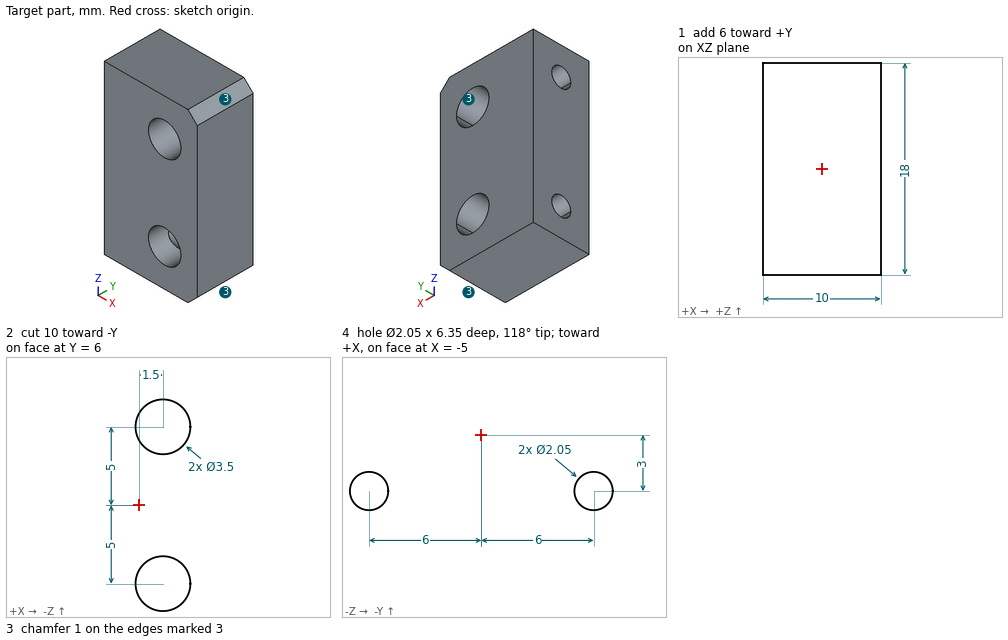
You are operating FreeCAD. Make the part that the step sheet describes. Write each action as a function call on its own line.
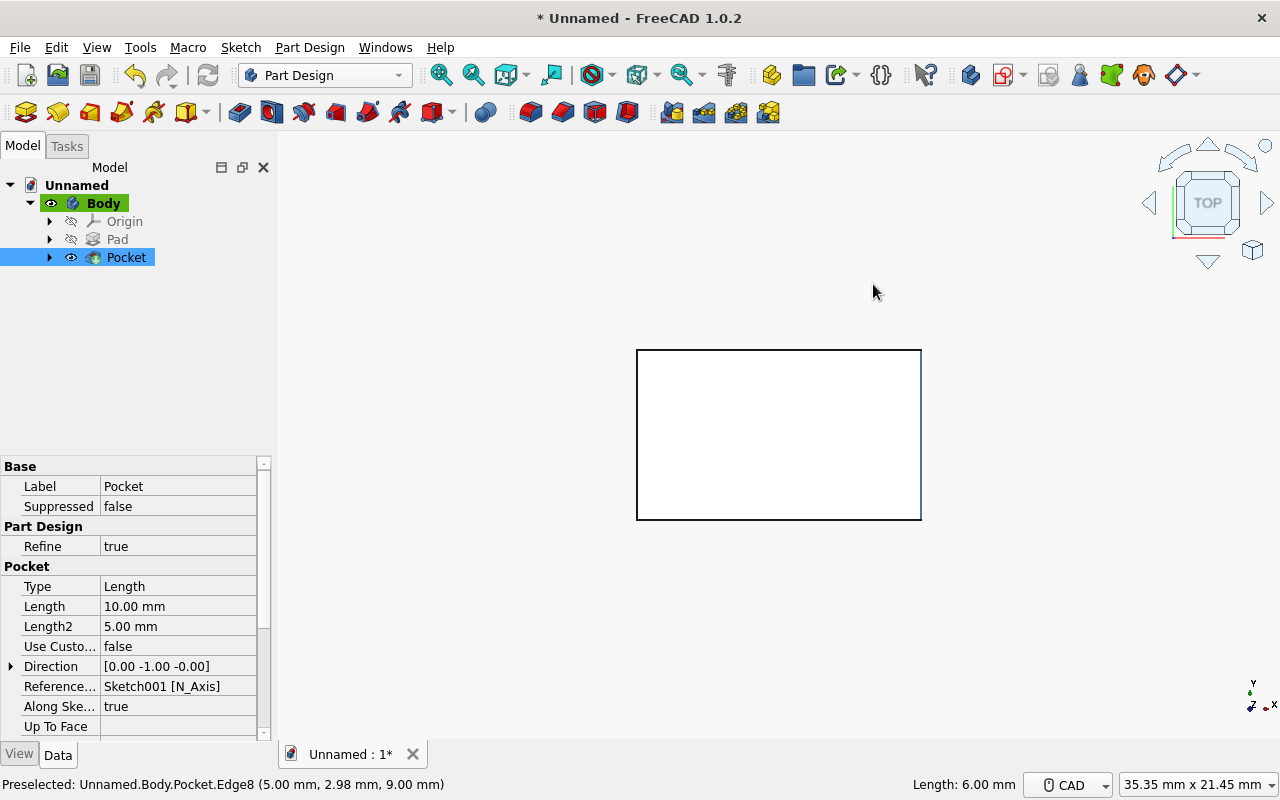
key(1)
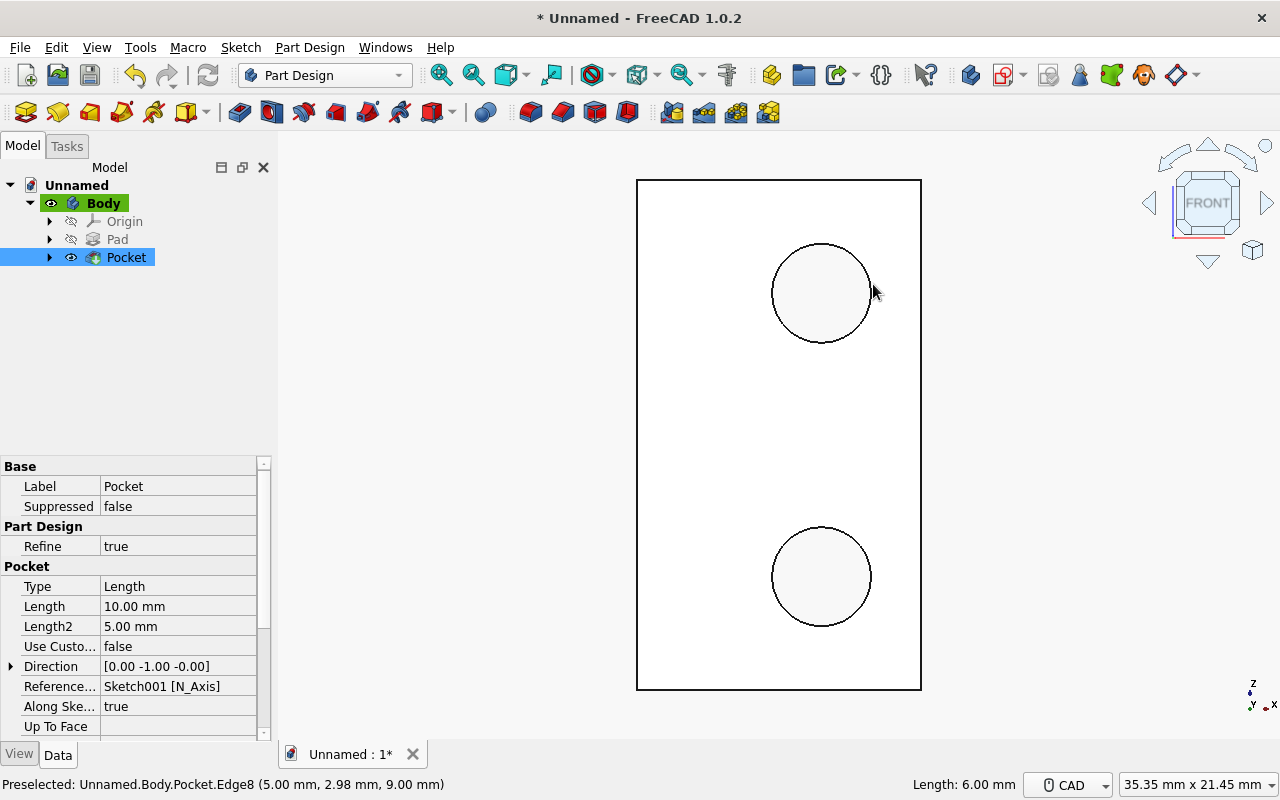
key(3)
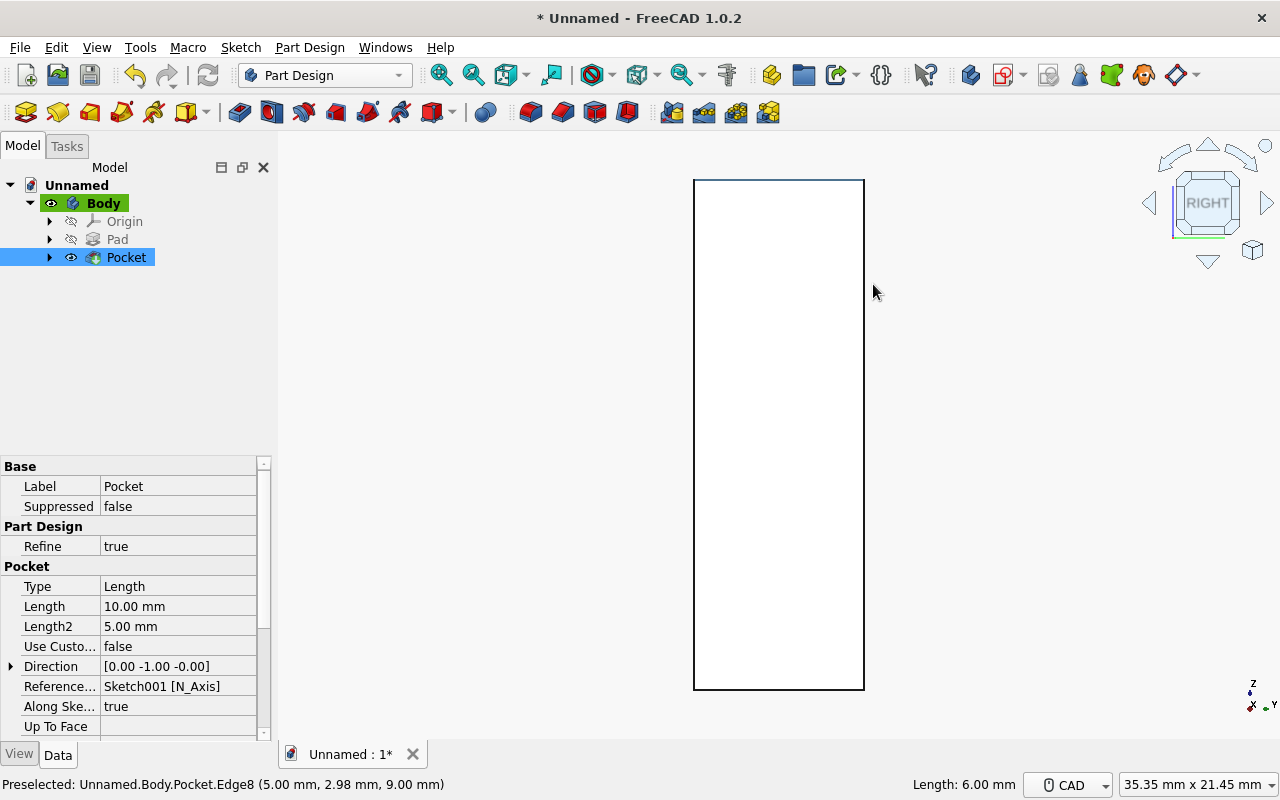
click(779, 689, ctrl)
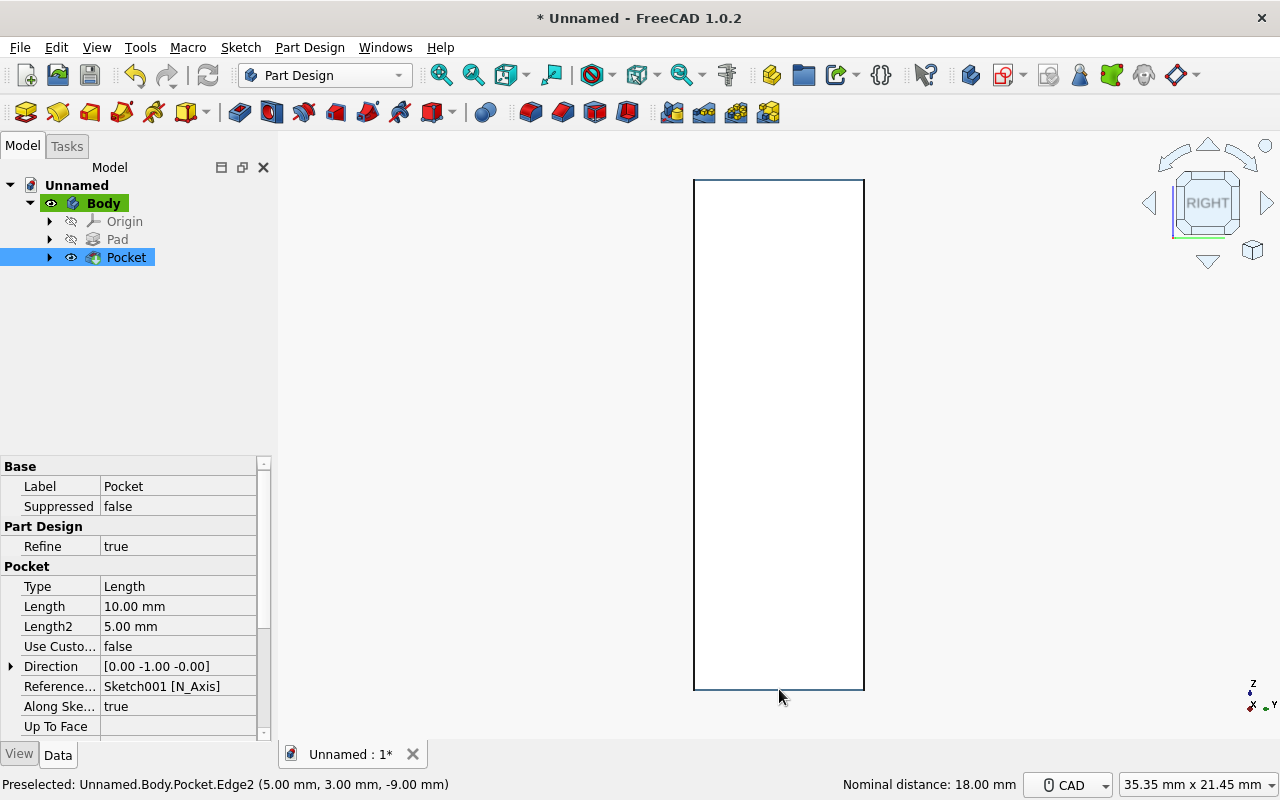
click(564, 112)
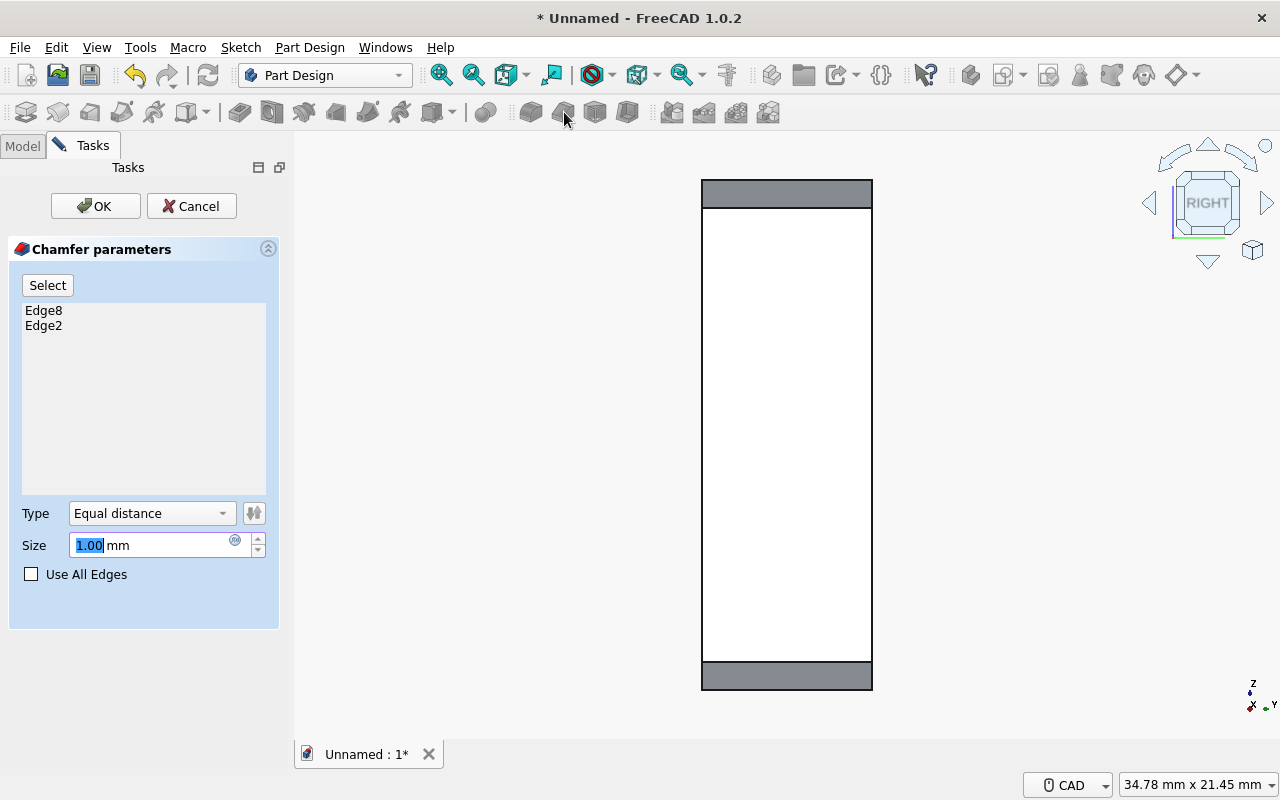
text(1)
key(Tab)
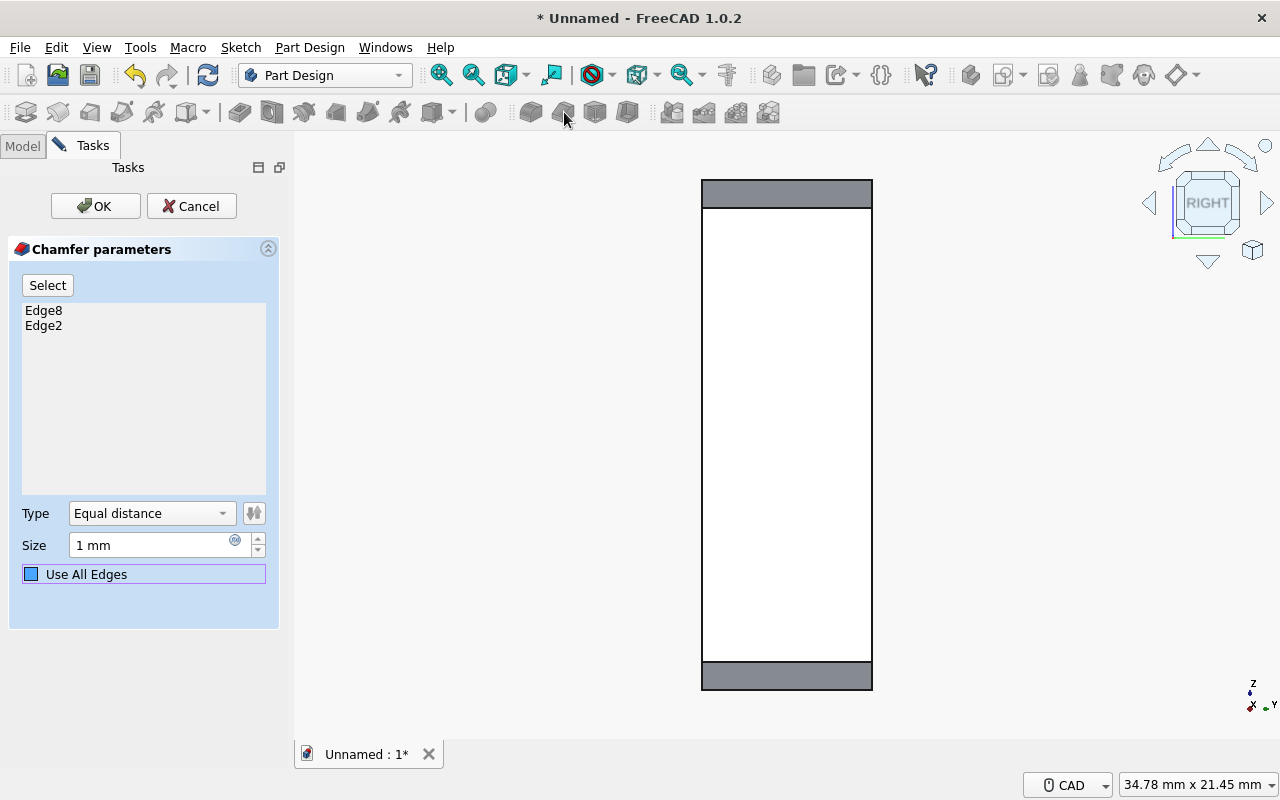
click(96, 206)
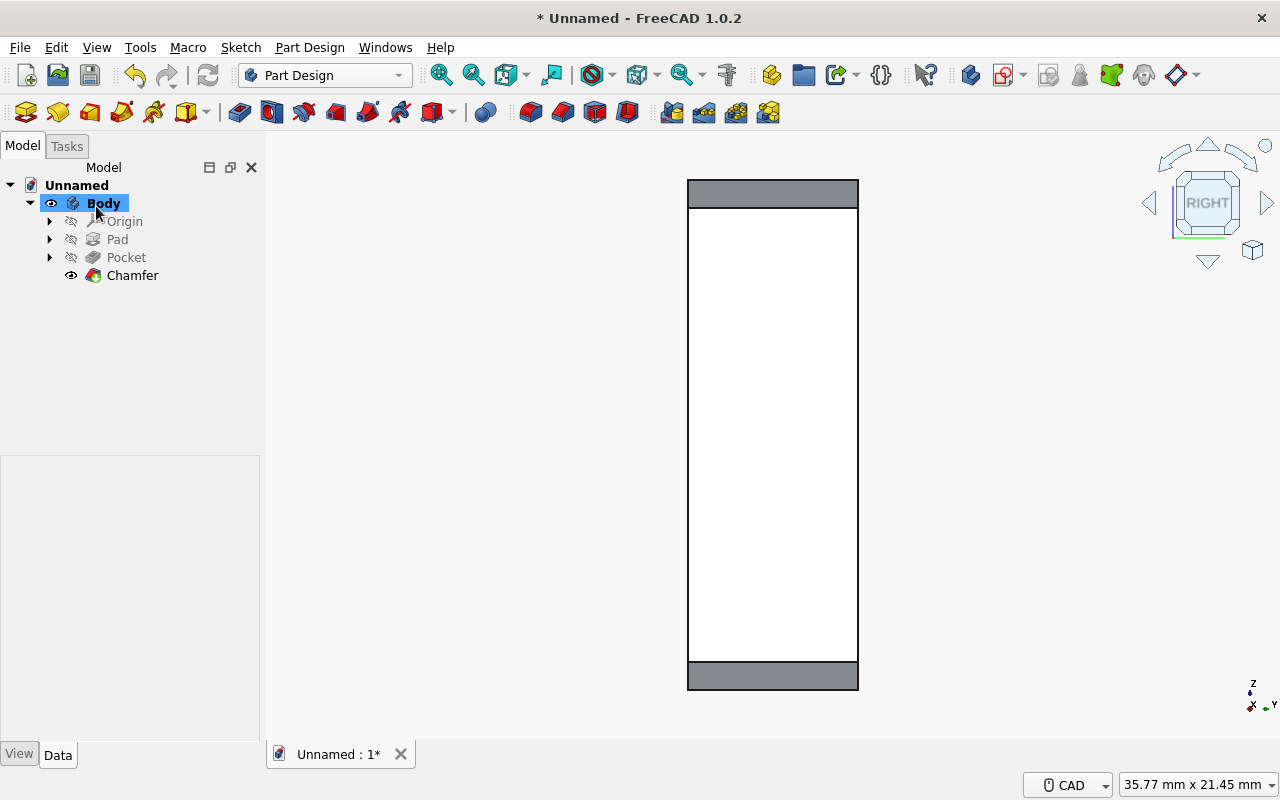
key(6)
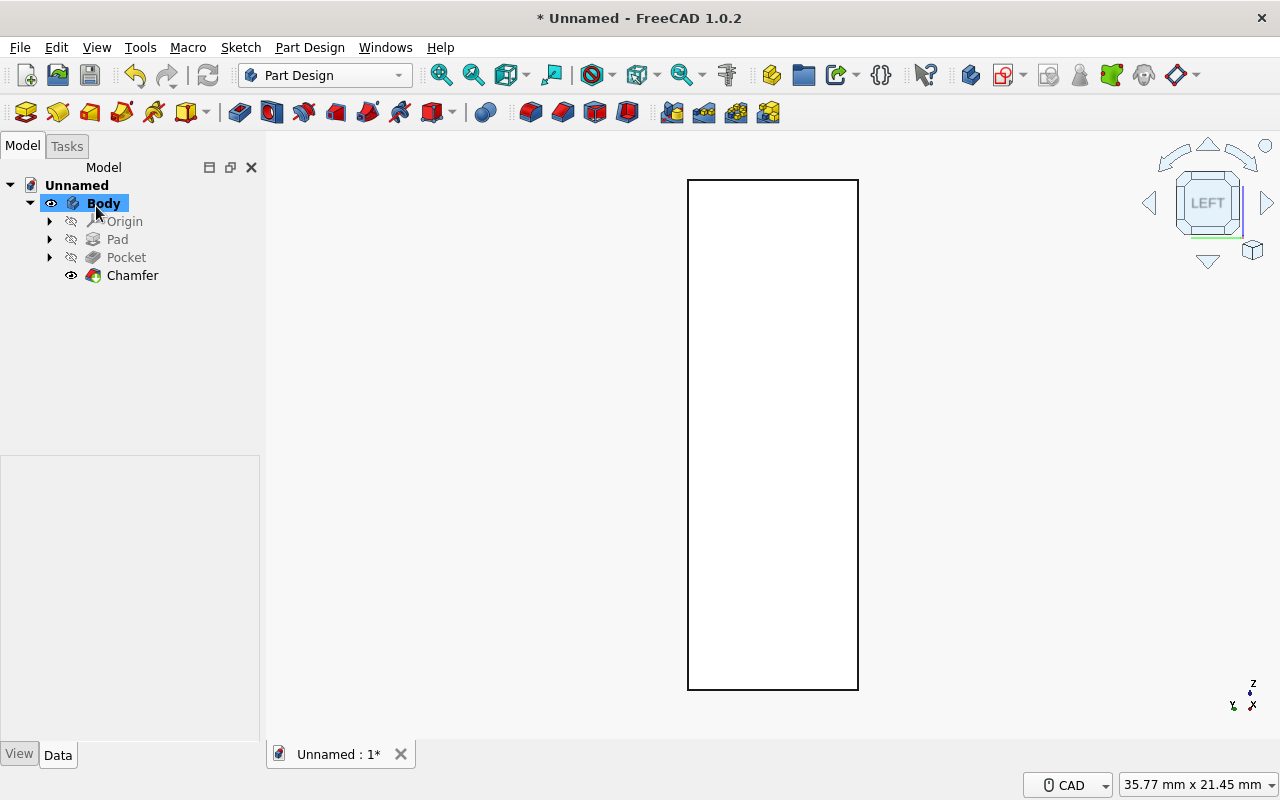
click(773, 434)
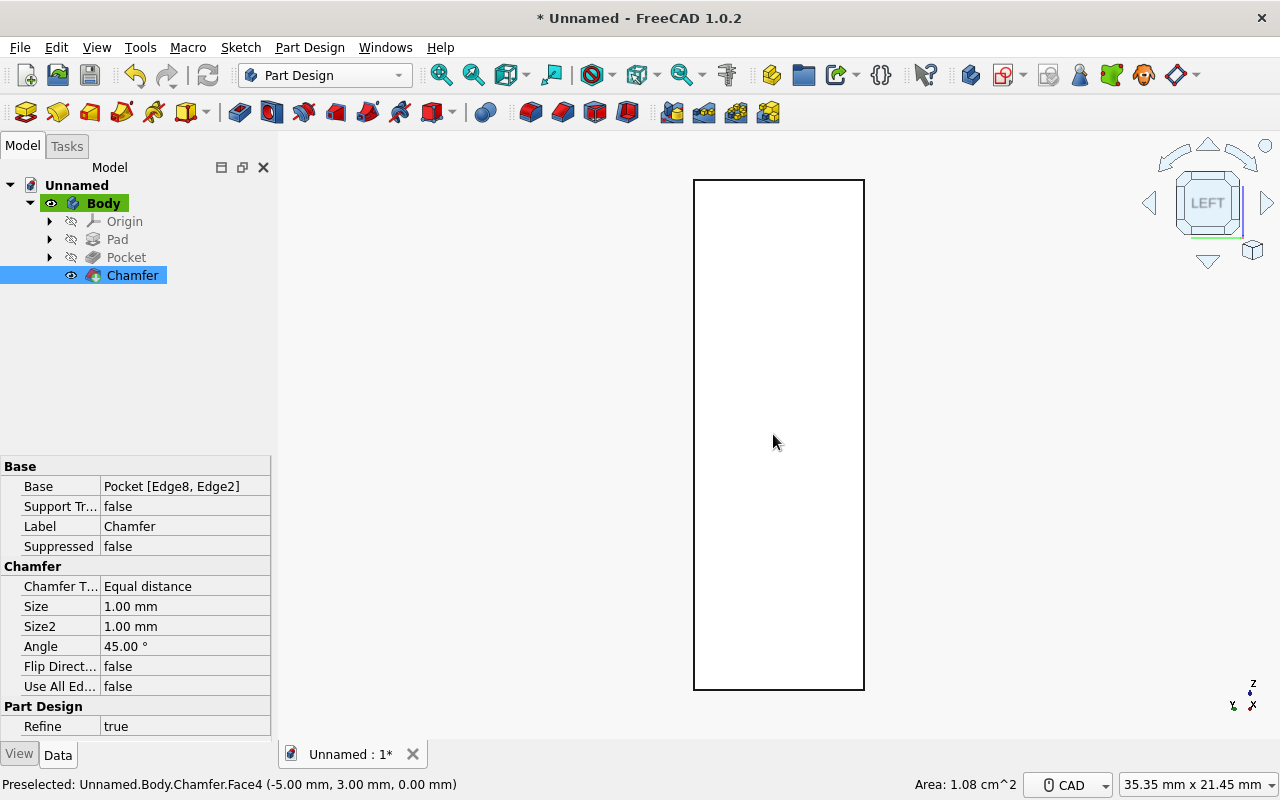
click(1004, 76)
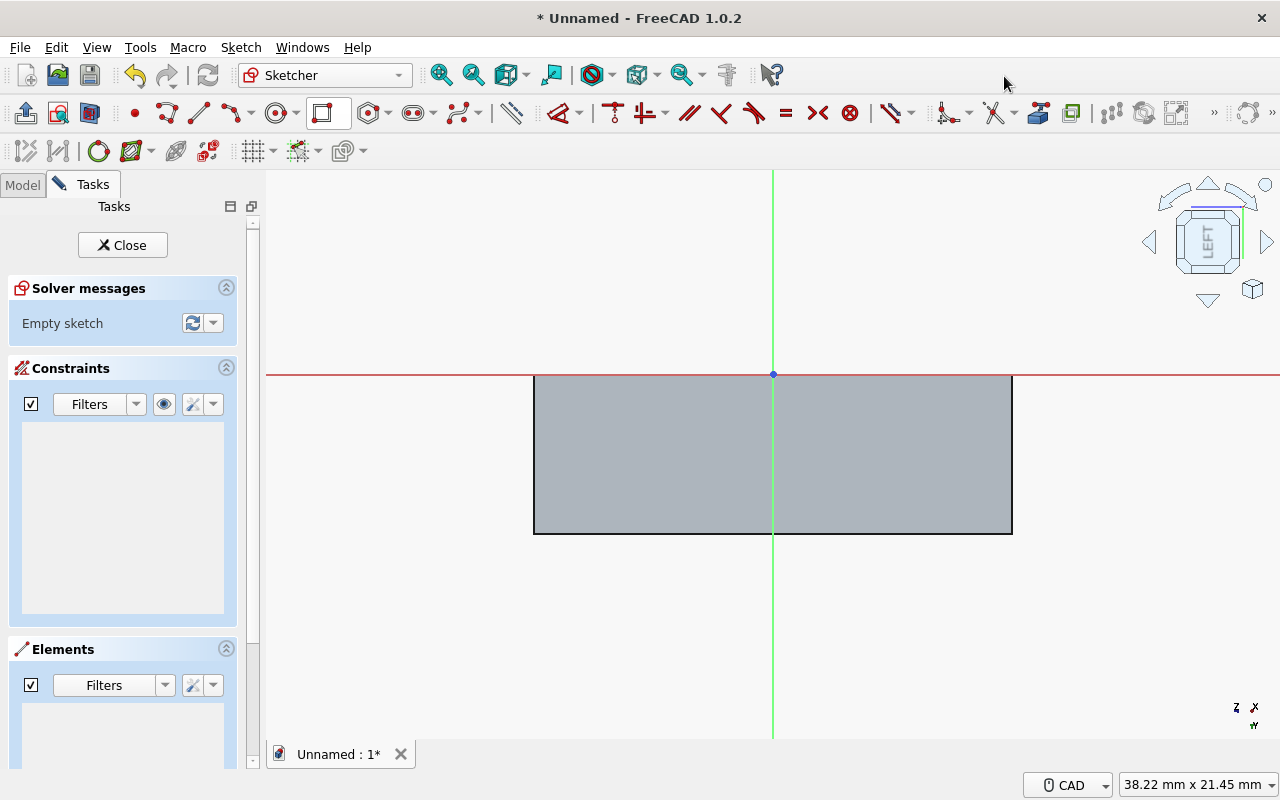
scroll(912, 375, up, 2)